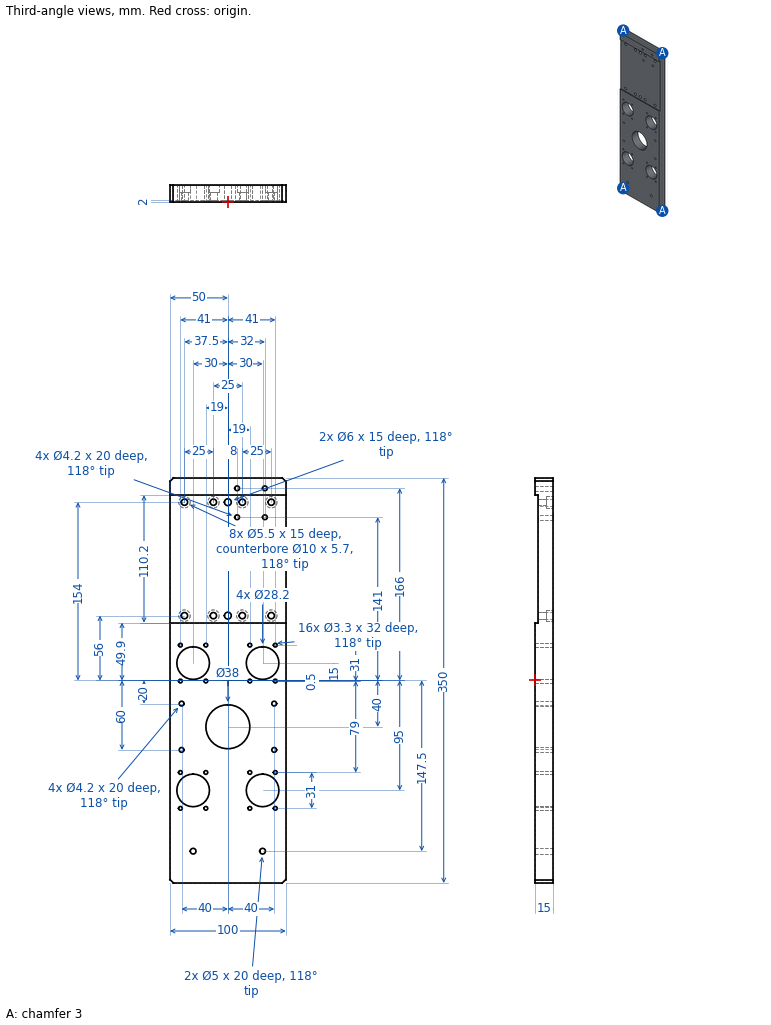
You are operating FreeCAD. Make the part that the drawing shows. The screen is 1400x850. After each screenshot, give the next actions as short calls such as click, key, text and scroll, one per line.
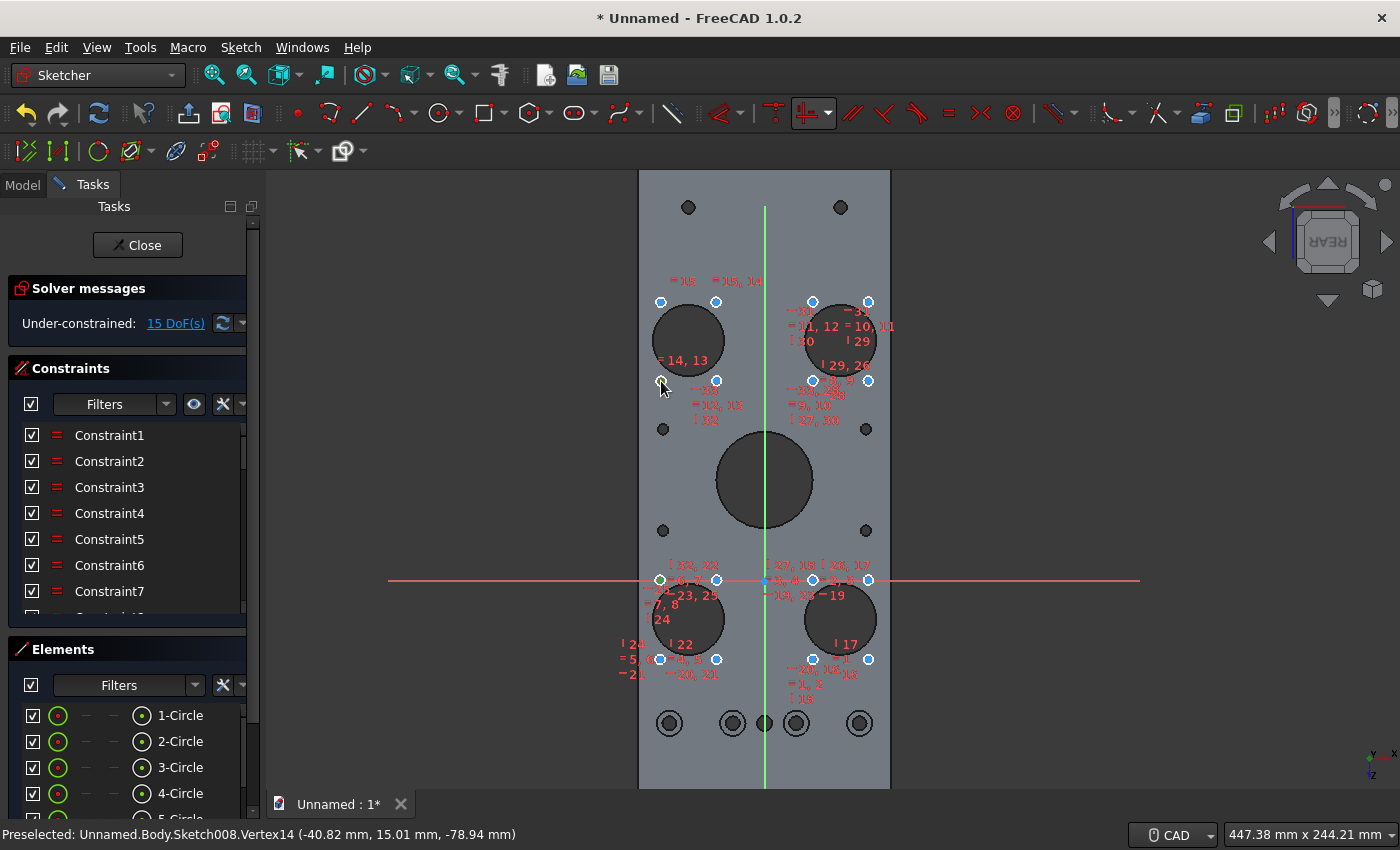
key(v)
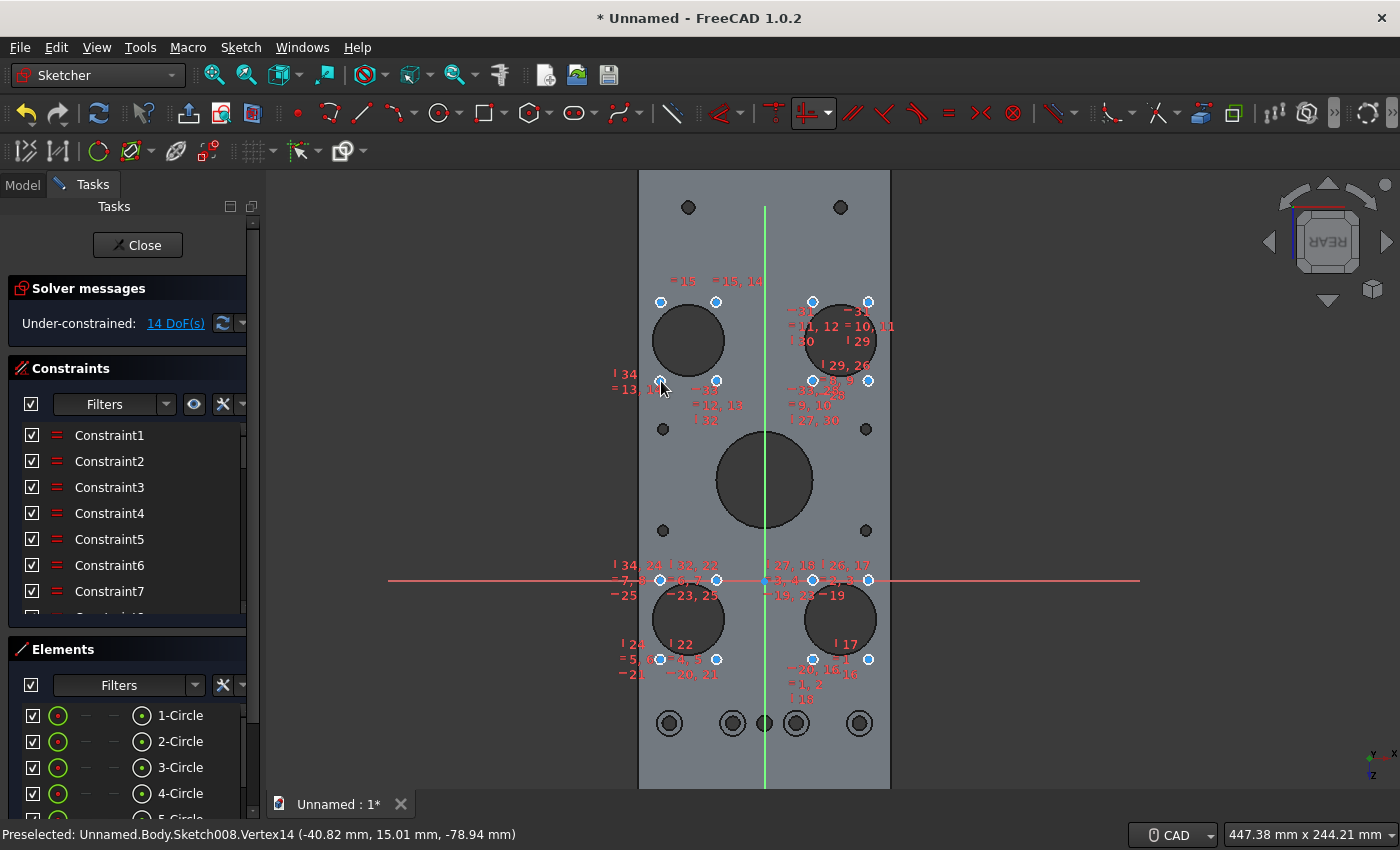
click(717, 381)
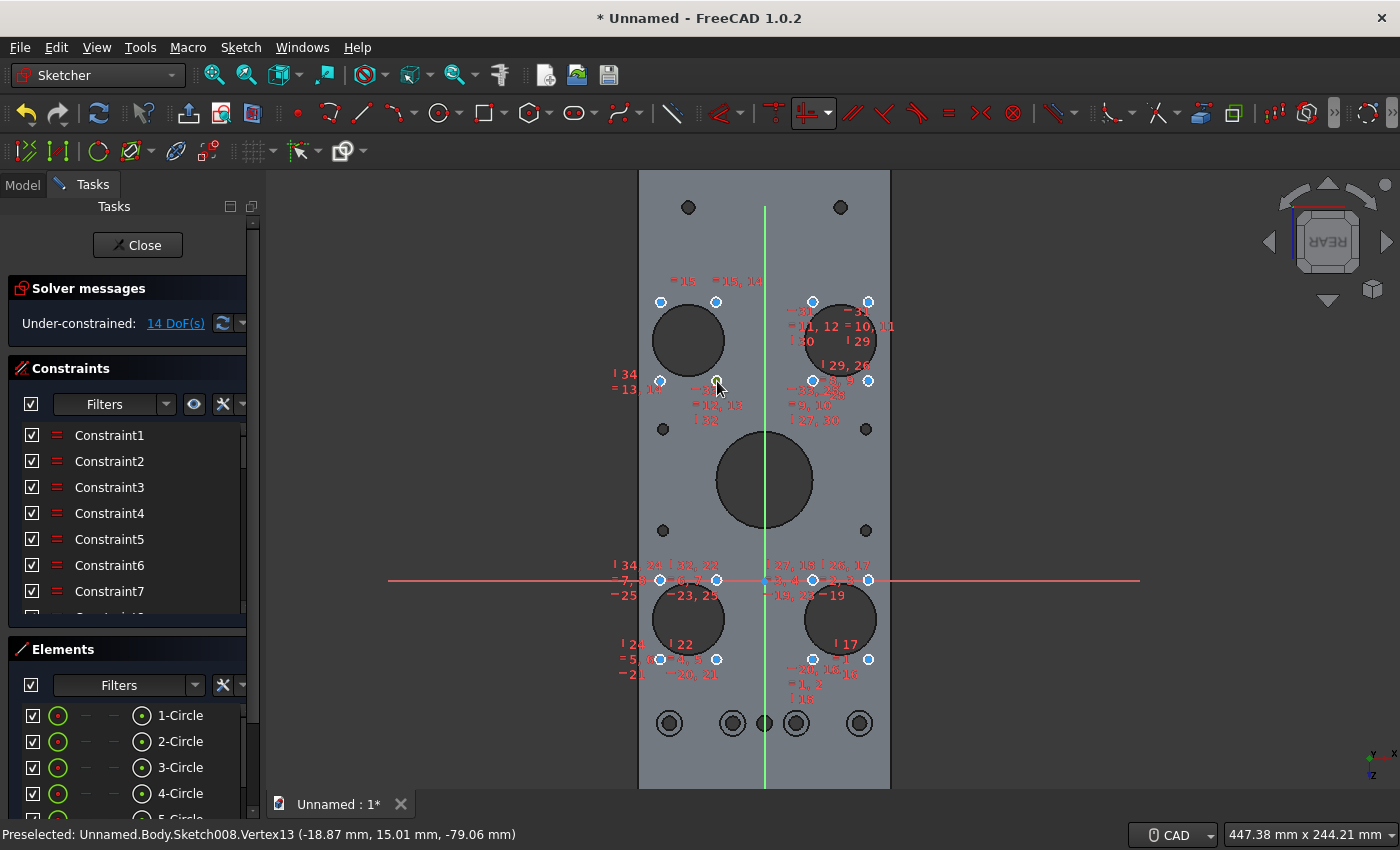
click(662, 383)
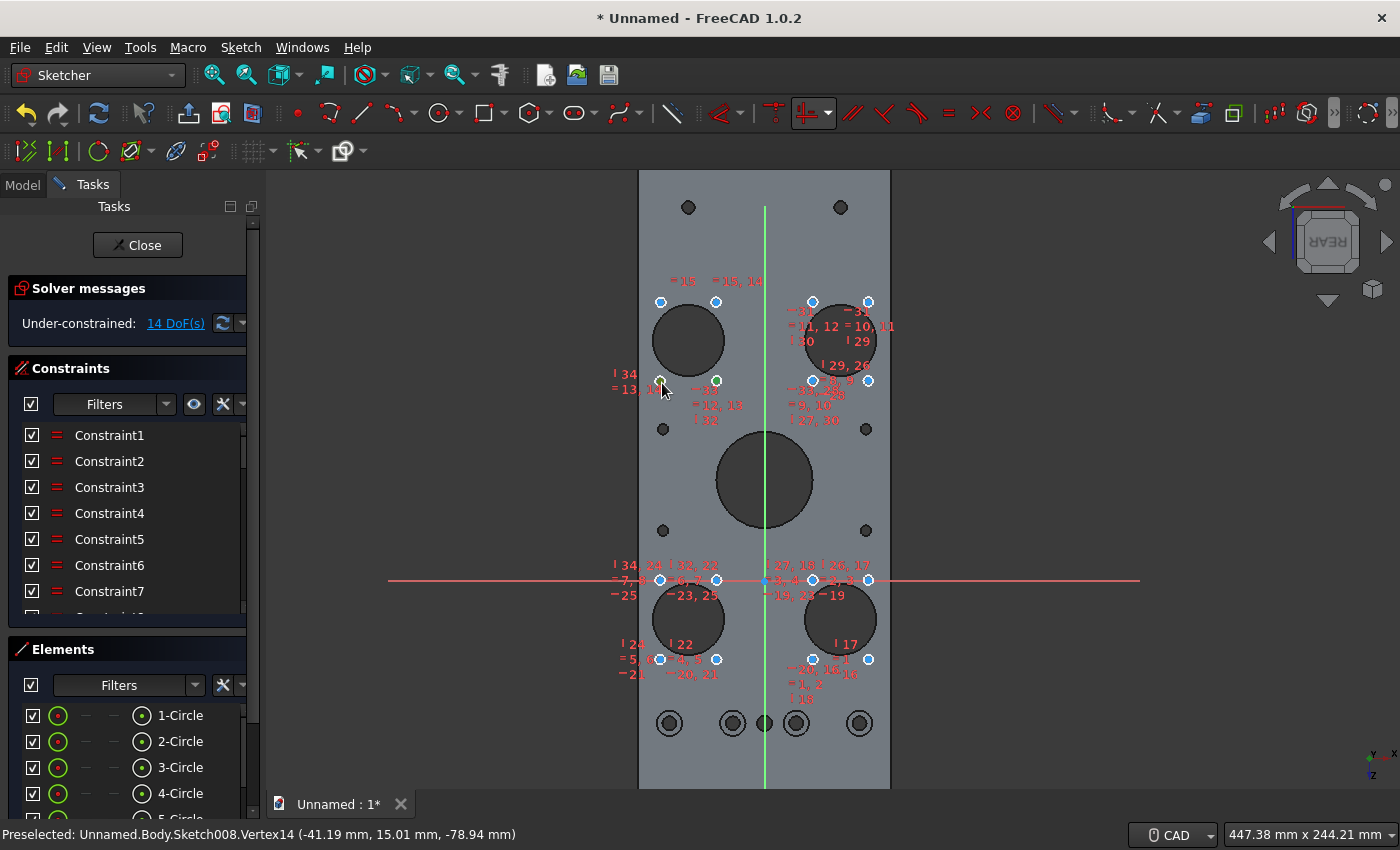
key(h)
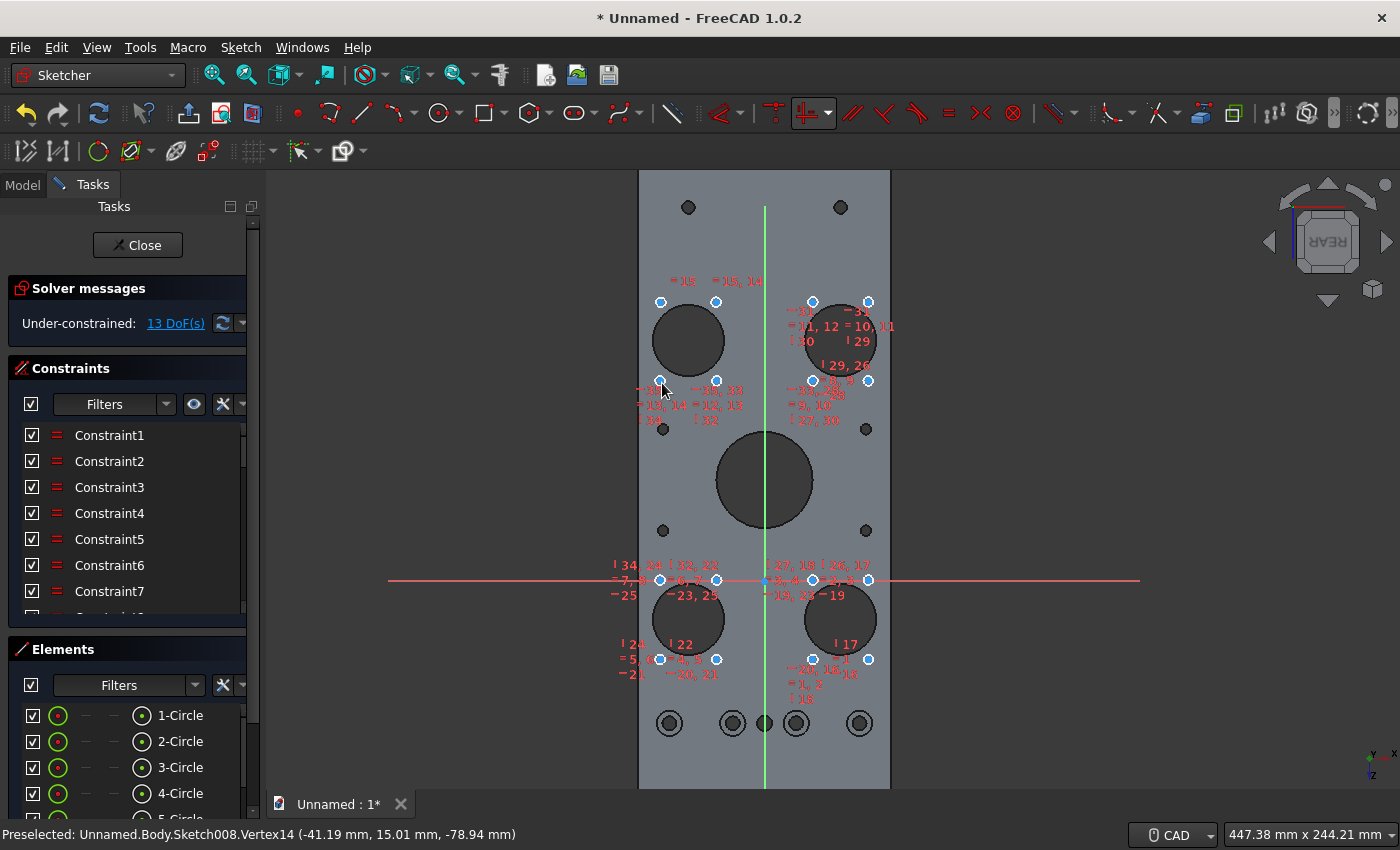
click(717, 381)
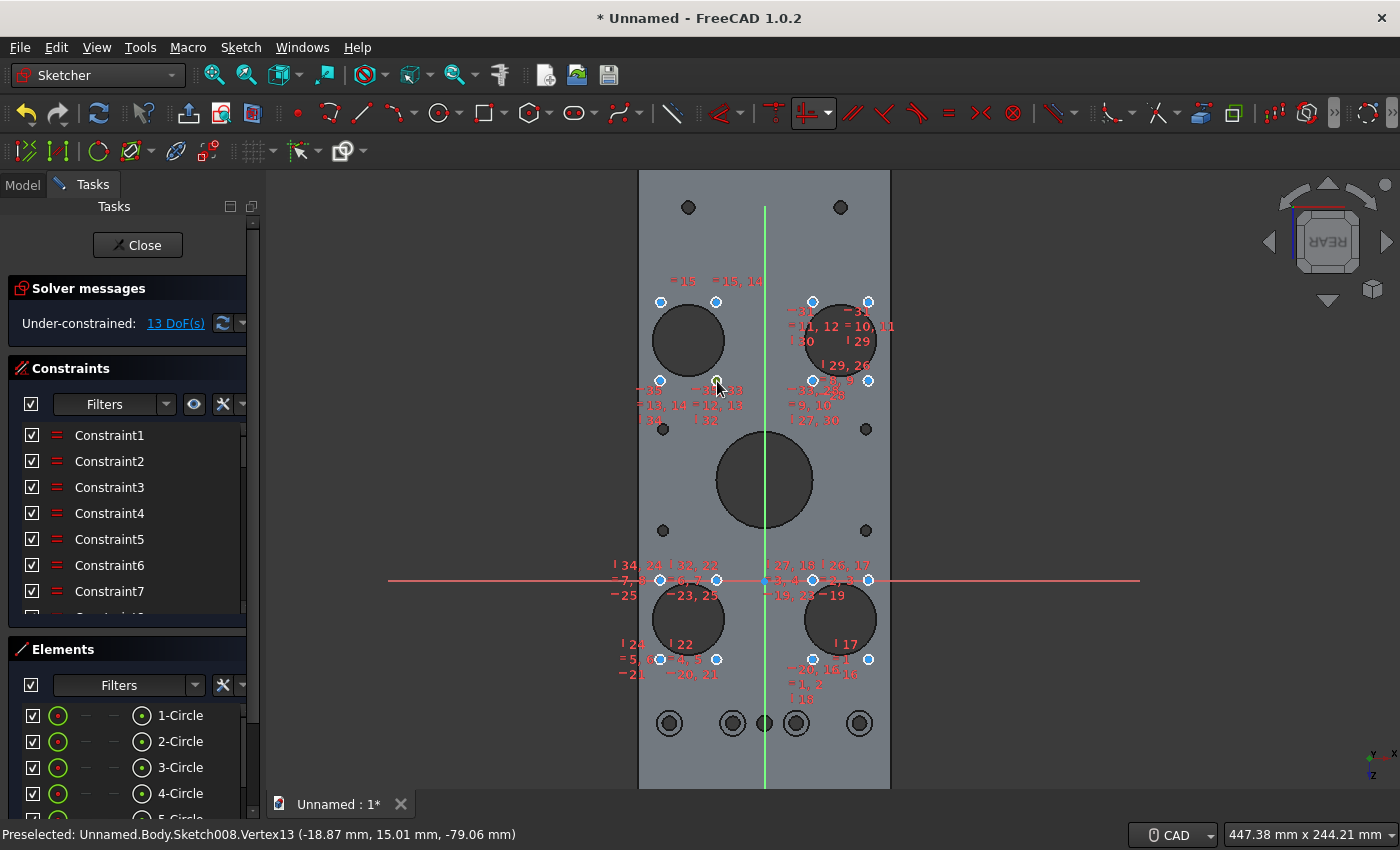
click(716, 302)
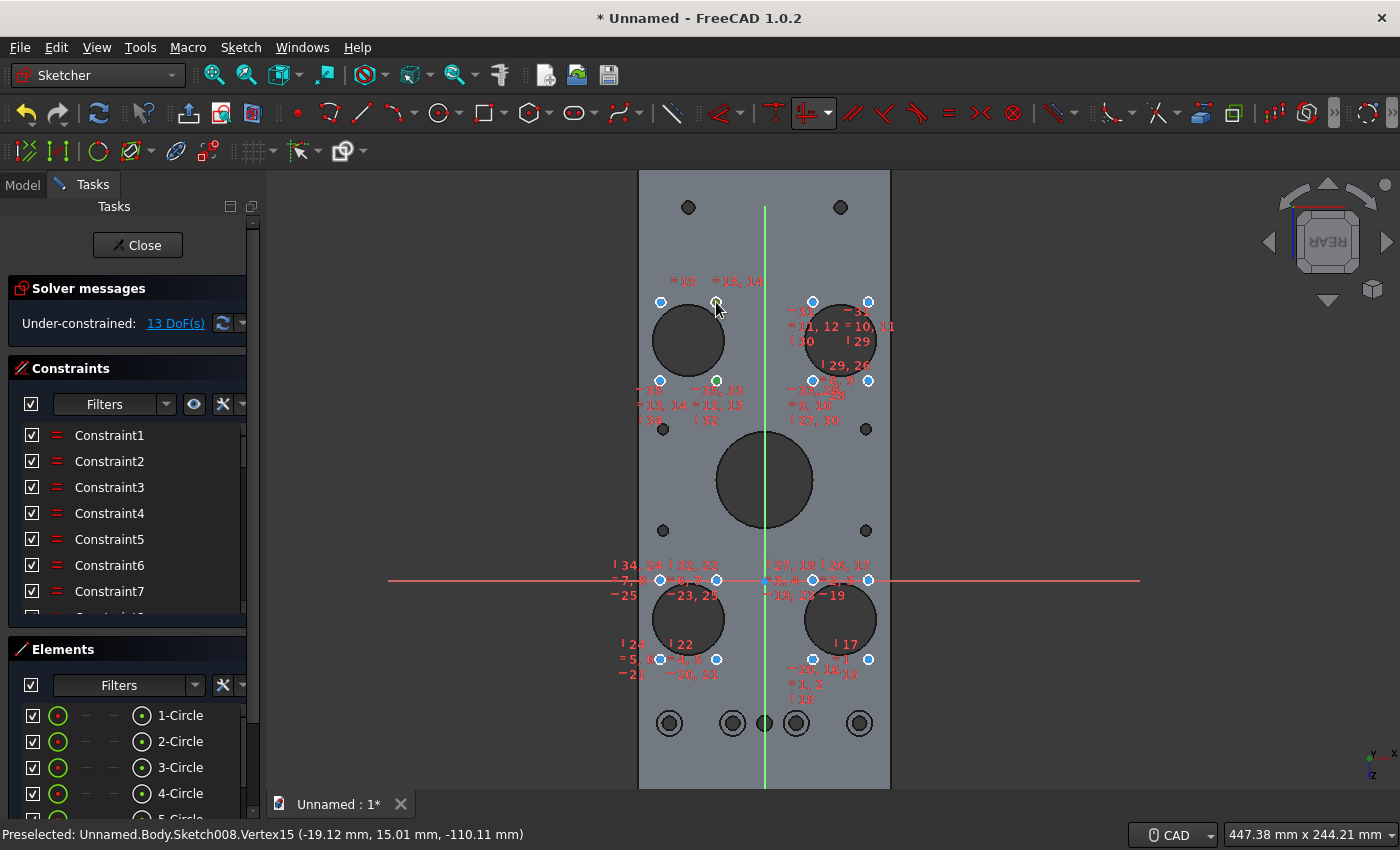
key(v)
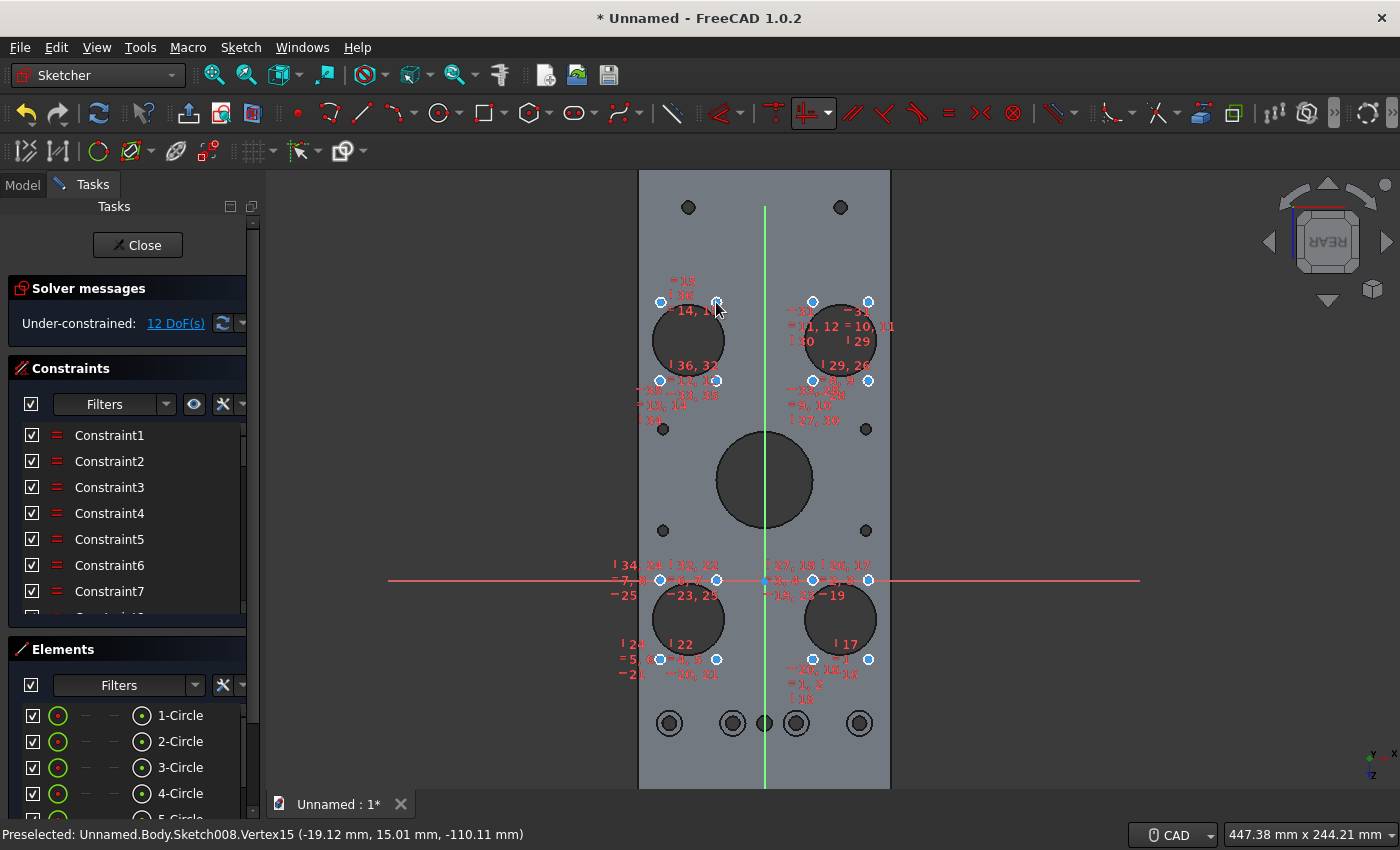
click(813, 302)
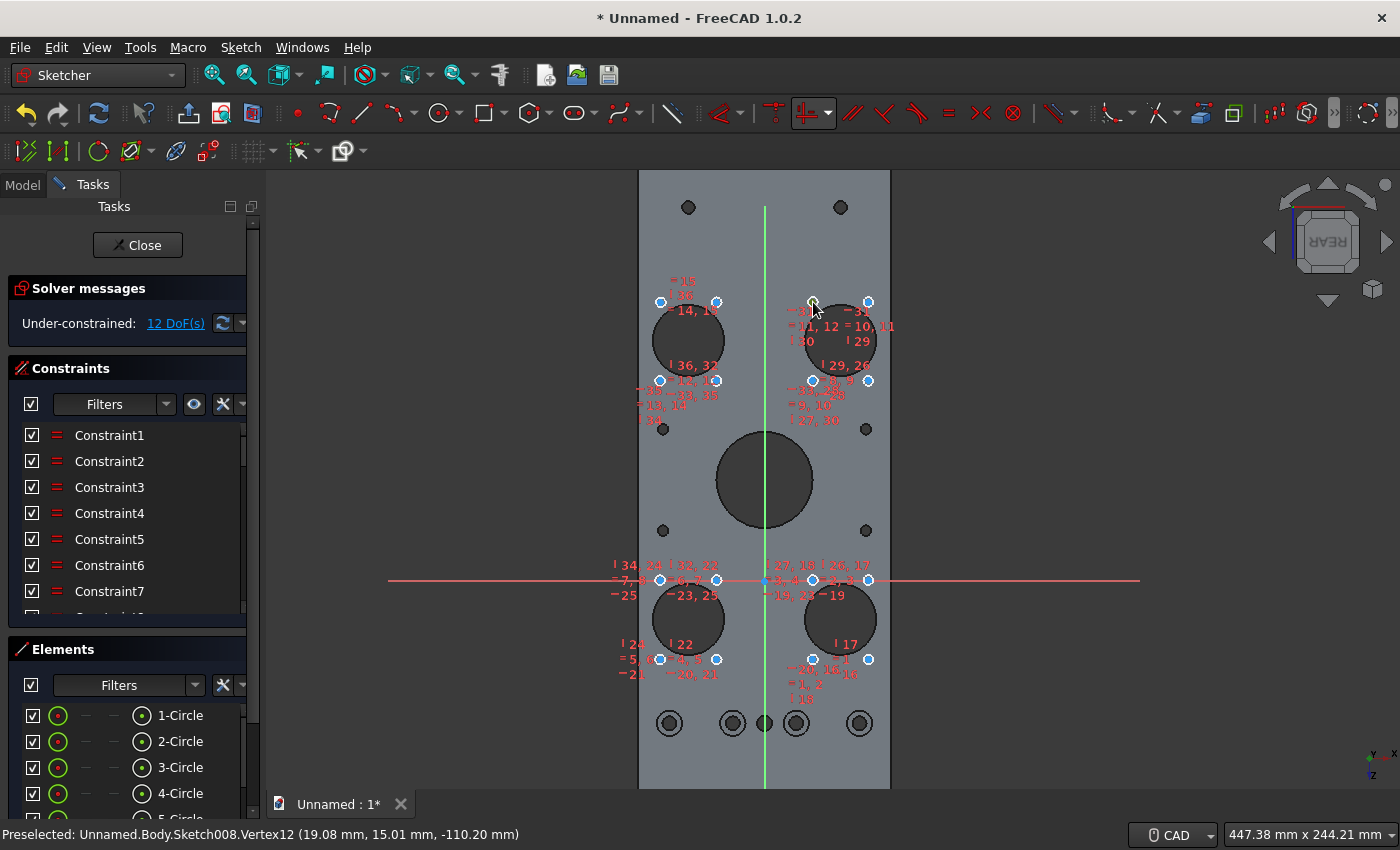
click(719, 304)